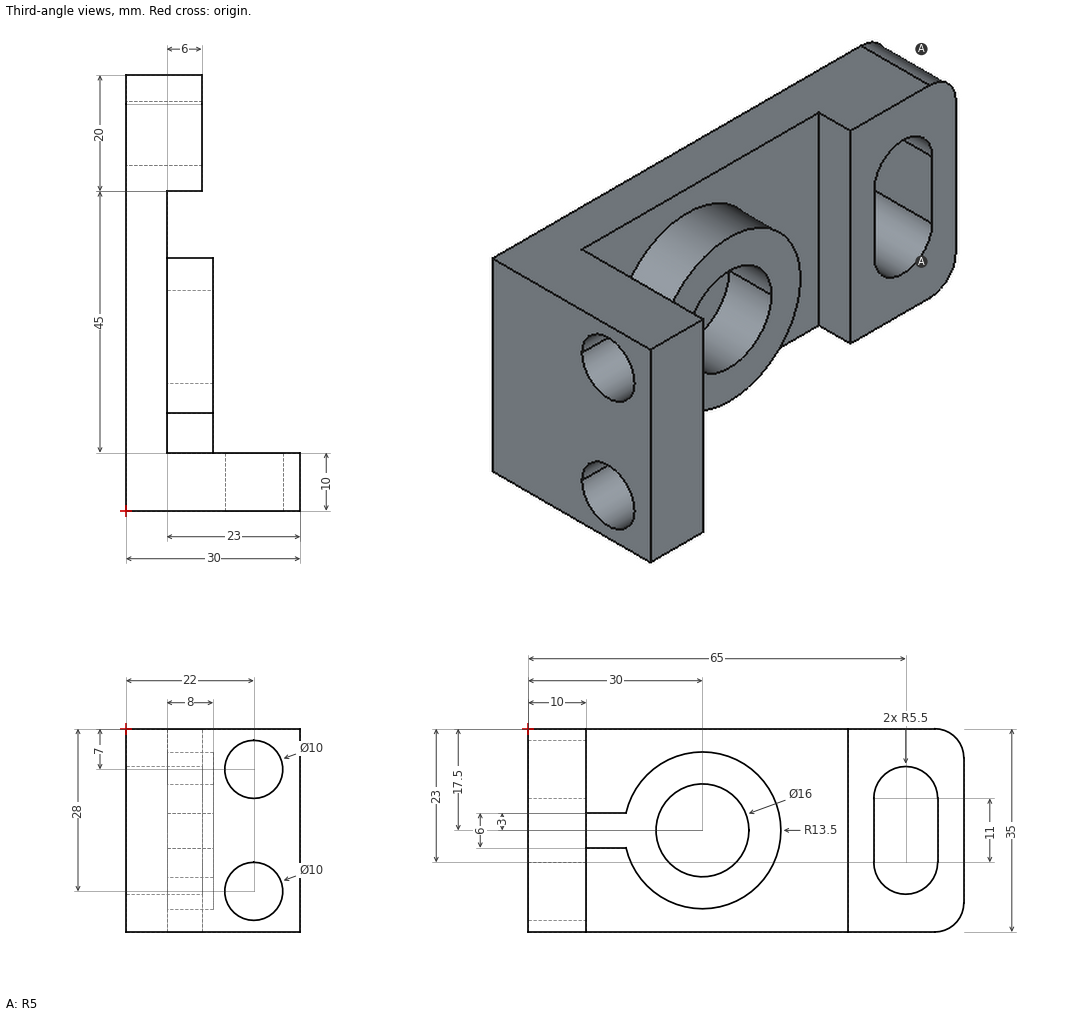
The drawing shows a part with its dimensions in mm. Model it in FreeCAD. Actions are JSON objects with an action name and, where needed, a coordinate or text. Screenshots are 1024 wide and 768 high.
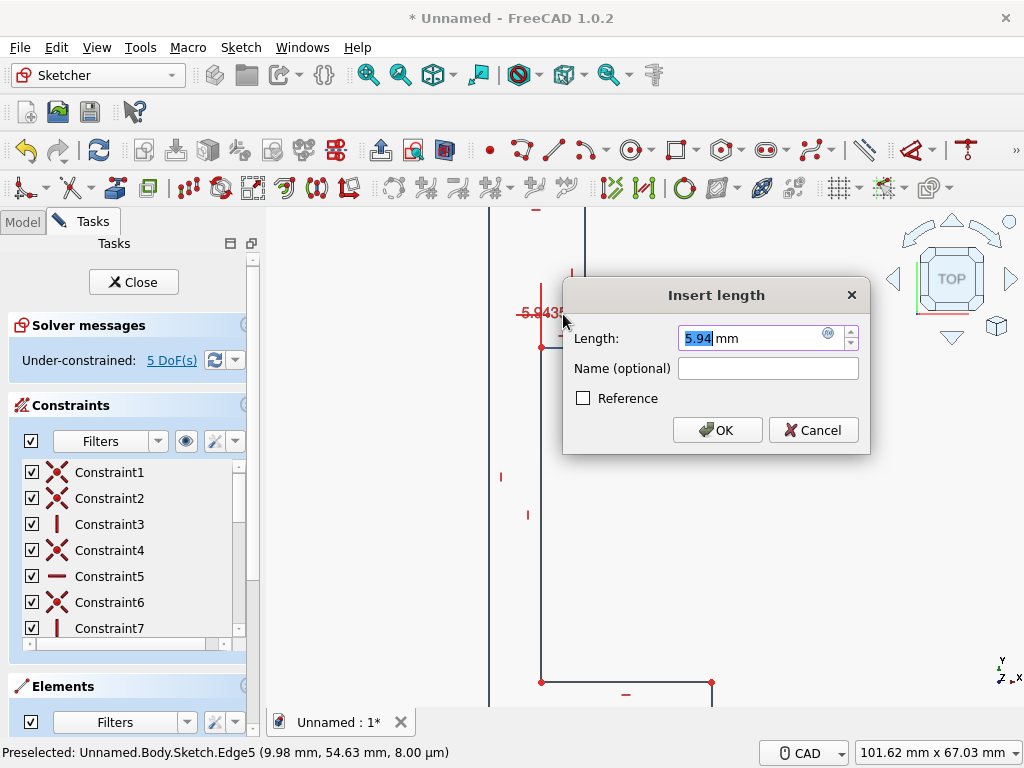
{"action": "type", "text": "6"}
{"action": "key", "text": "Return"}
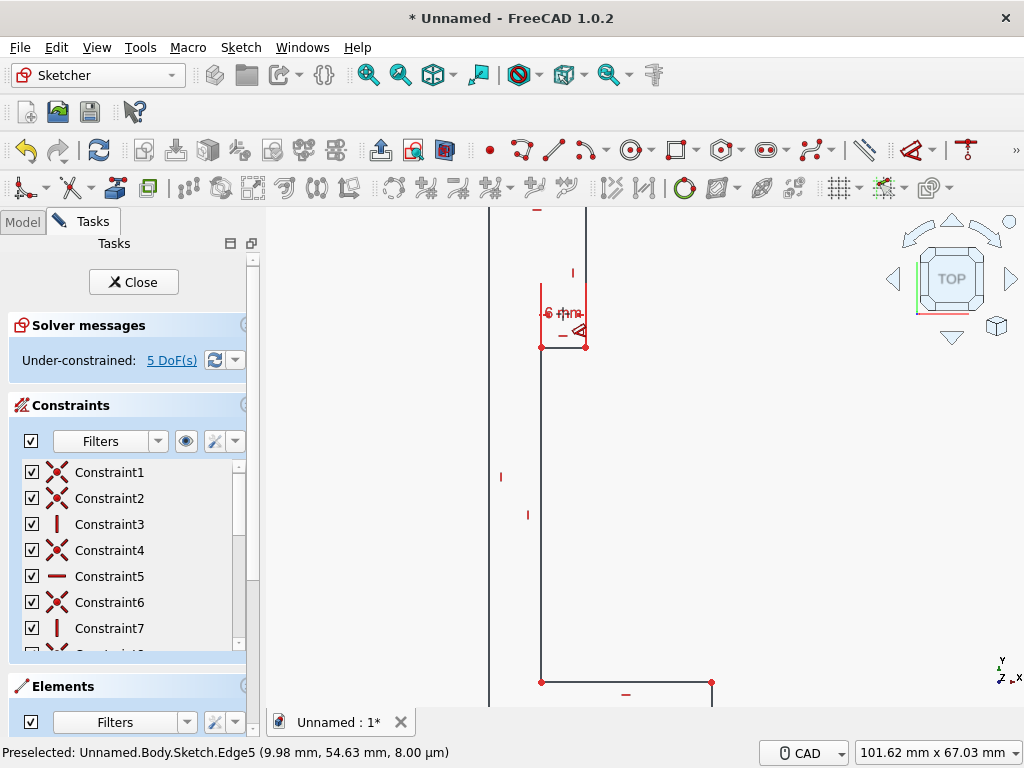
{"action": "scroll", "coordinate": [547, 435], "scroll_direction": "down", "scroll_amount": 3}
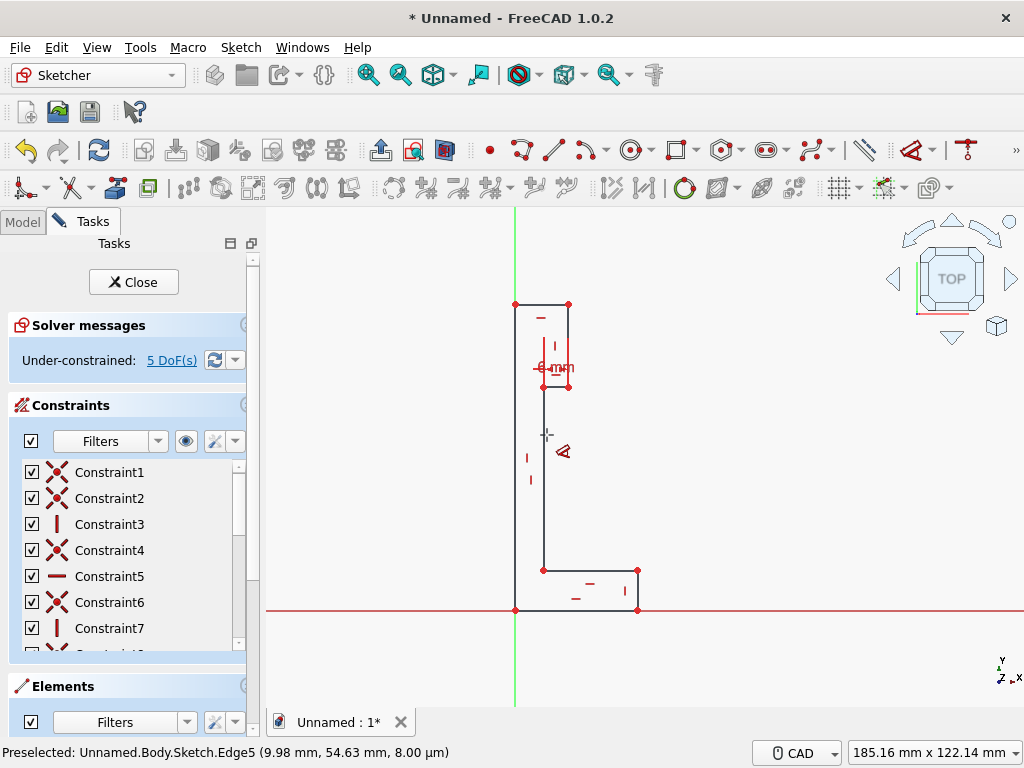
{"action": "left_click", "coordinate": [552, 611]}
{"action": "left_click", "coordinate": [576, 645]}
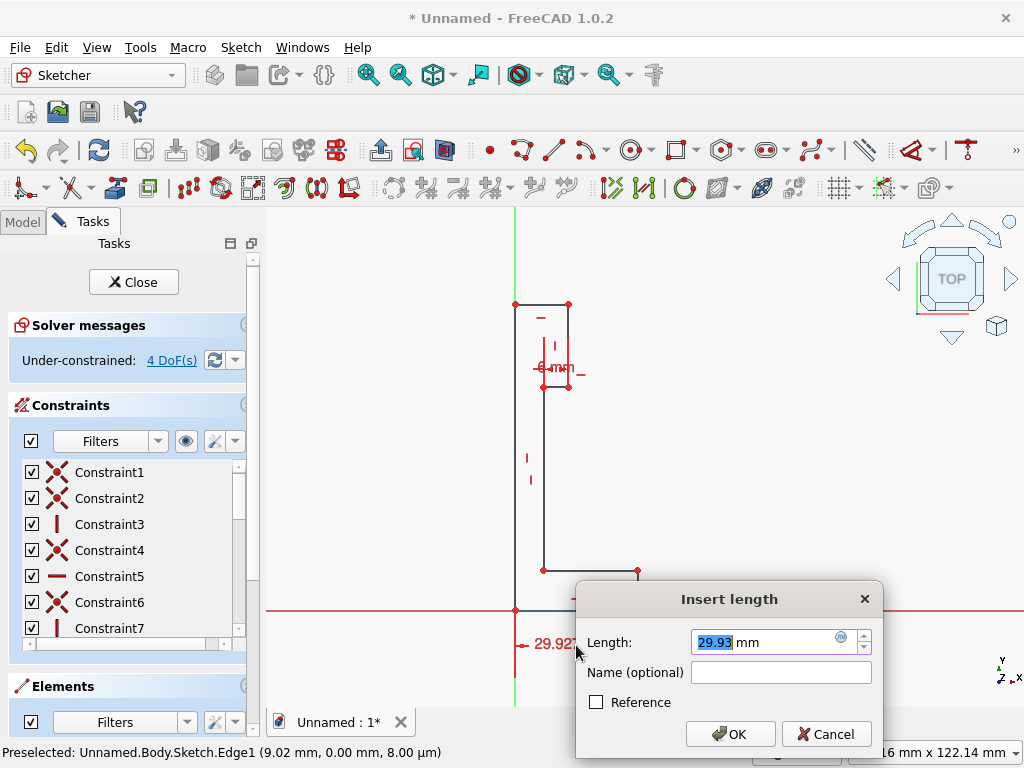
{"action": "type", "text": "30"}
{"action": "key", "text": "Return"}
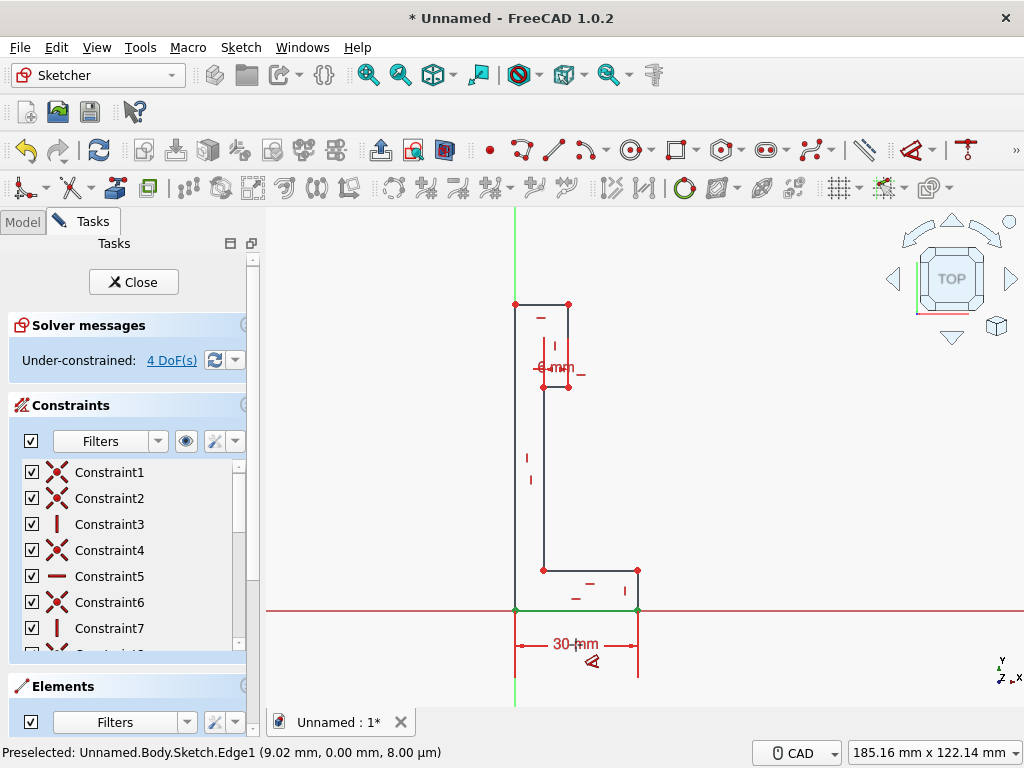
{"action": "left_click", "coordinate": [638, 599]}
{"action": "left_click", "coordinate": [672, 591]}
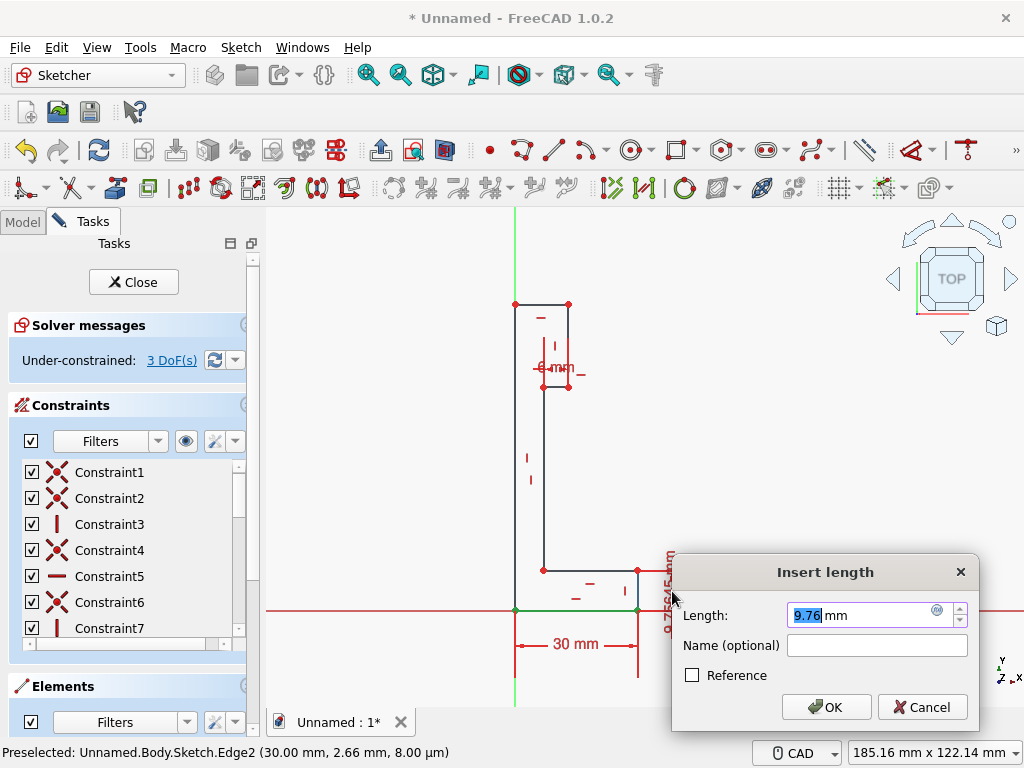
{"action": "type", "text": "10"}
{"action": "key", "text": "Return"}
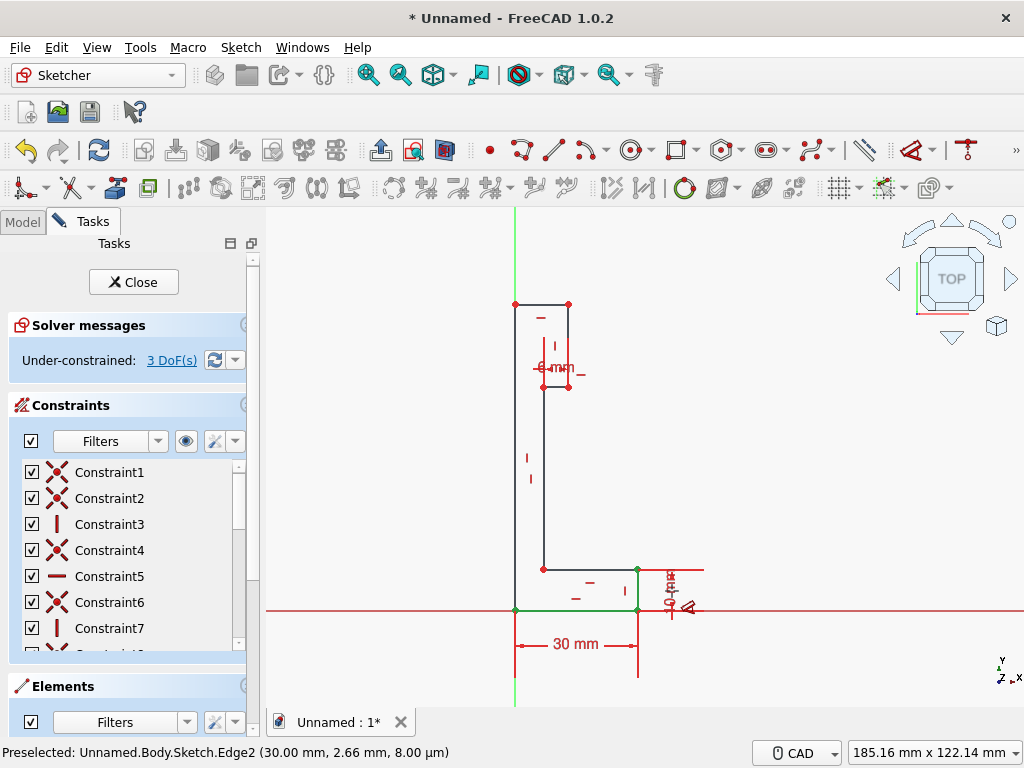
{"action": "left_click", "coordinate": [610, 570]}
{"action": "left_click", "coordinate": [591, 536]}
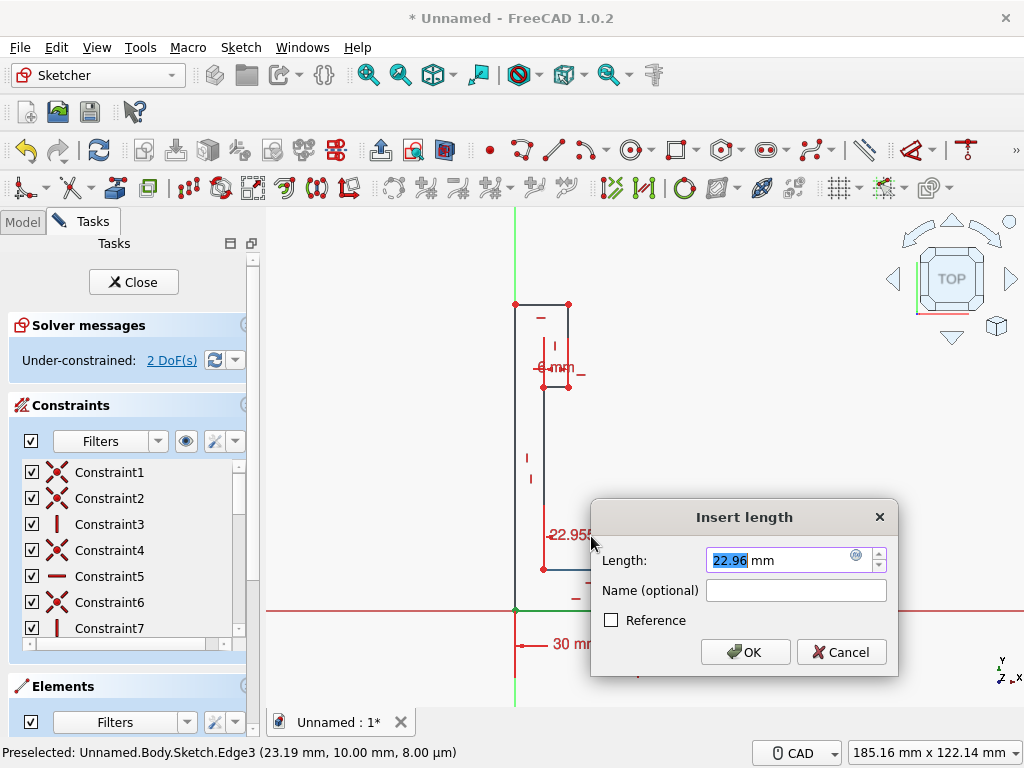
{"action": "type", "text": "23"}
{"action": "key", "text": "Return"}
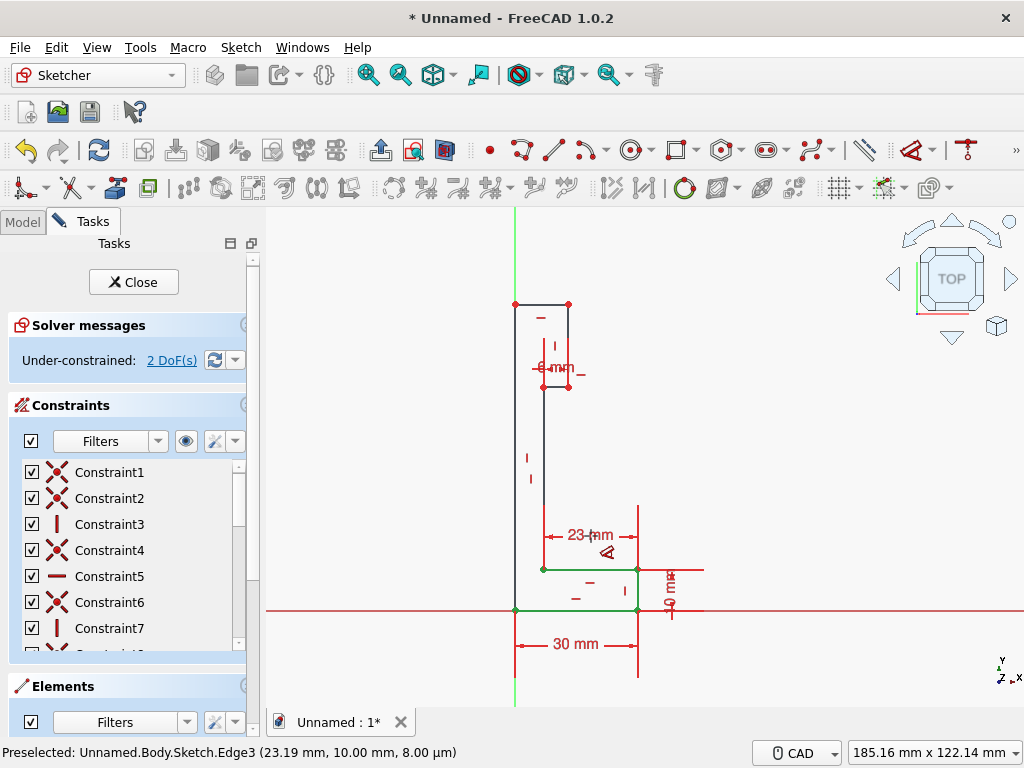
{"action": "left_click", "coordinate": [544, 515]}
{"action": "left_click", "coordinate": [578, 479]}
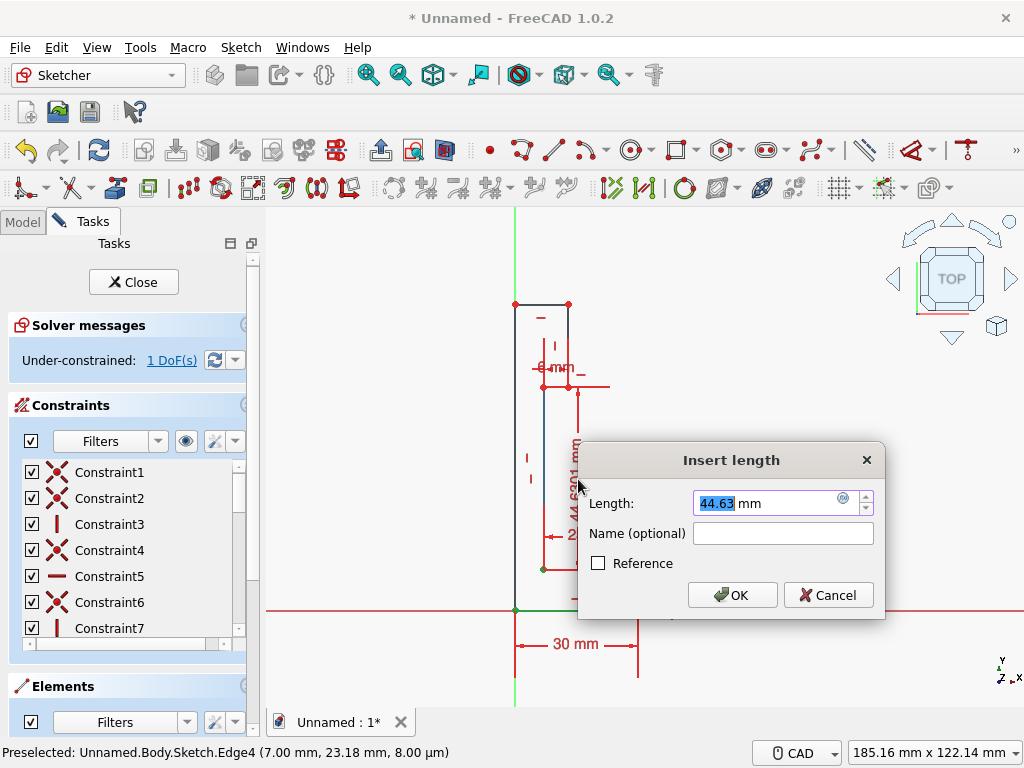
{"action": "type", "text": "45"}
{"action": "key", "text": "Return"}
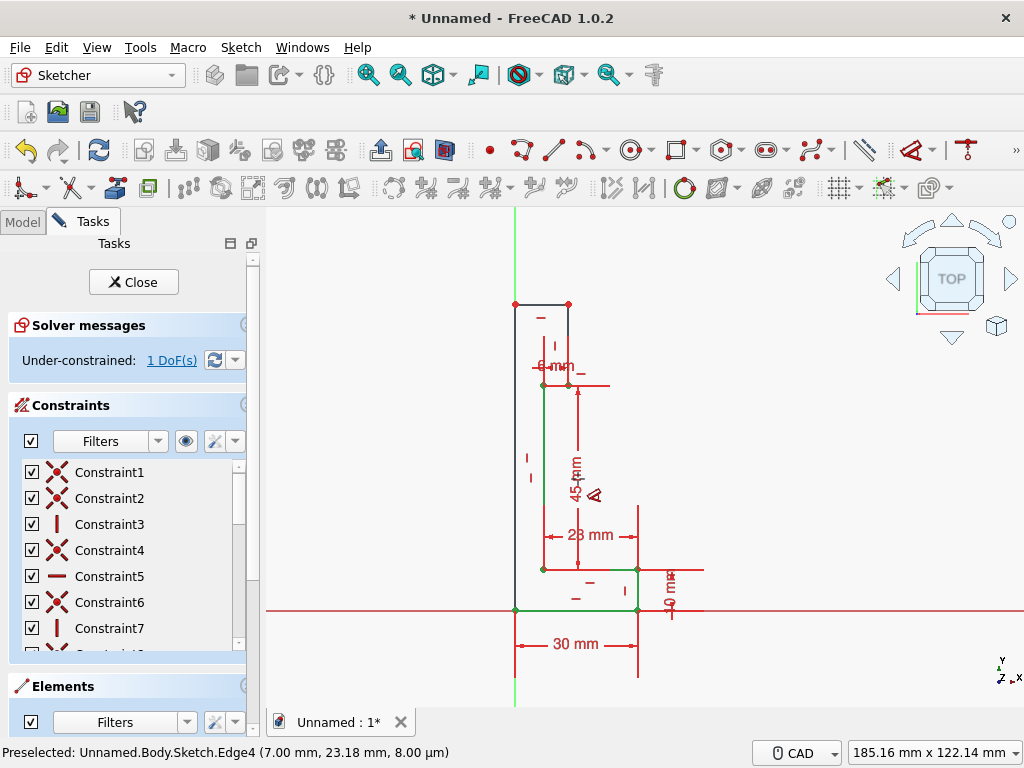
{"action": "left_click", "coordinate": [568, 361]}
{"action": "left_click", "coordinate": [534, 345]}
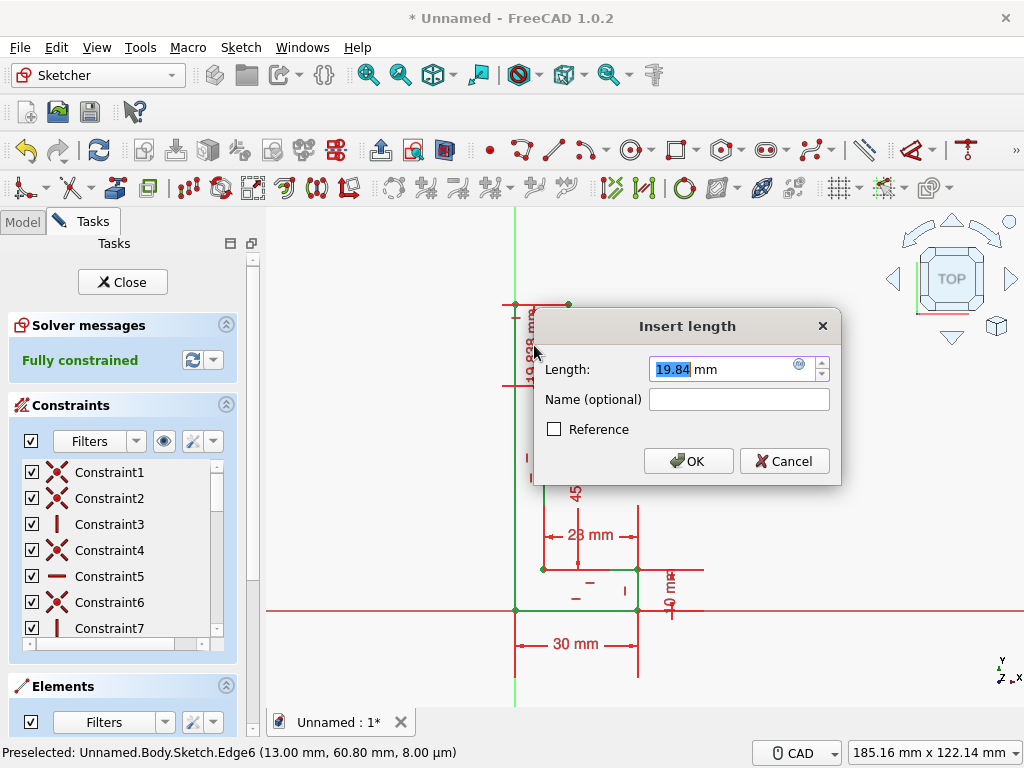
{"action": "type", "text": "20"}
{"action": "key", "text": "Return"}
{"action": "key", "text": "Escape"}